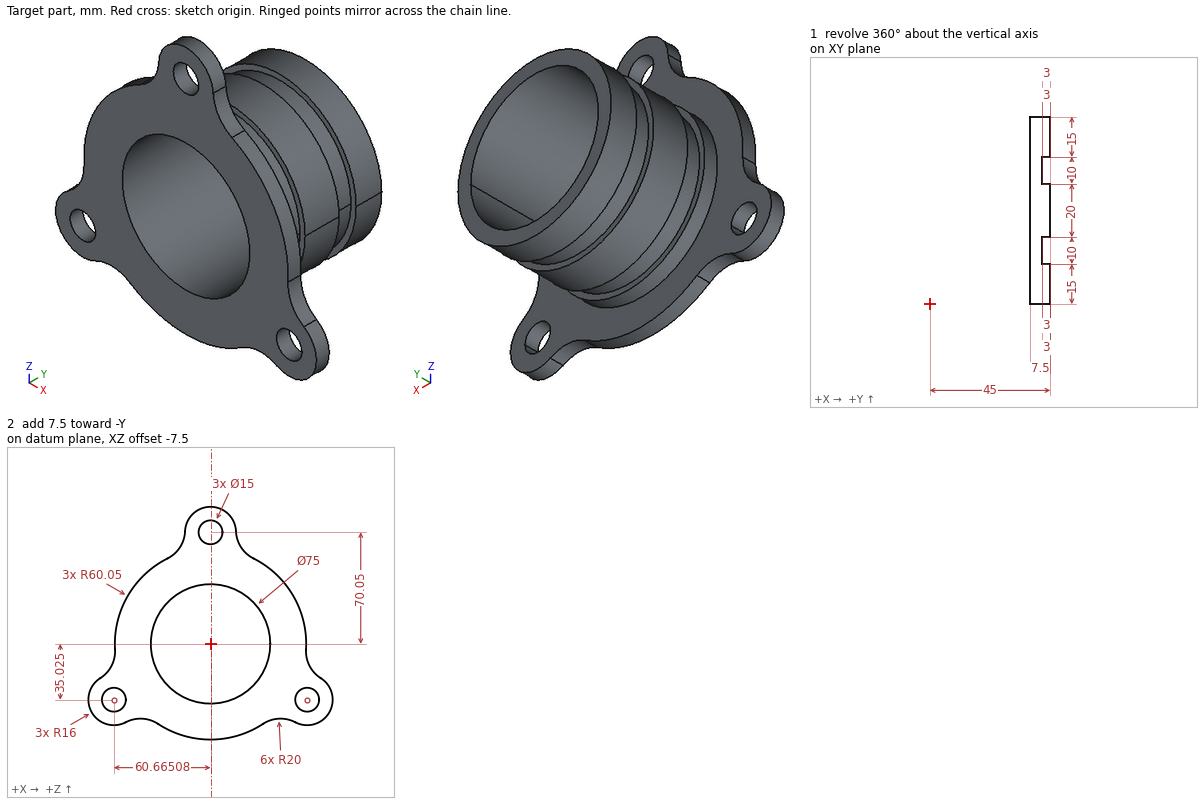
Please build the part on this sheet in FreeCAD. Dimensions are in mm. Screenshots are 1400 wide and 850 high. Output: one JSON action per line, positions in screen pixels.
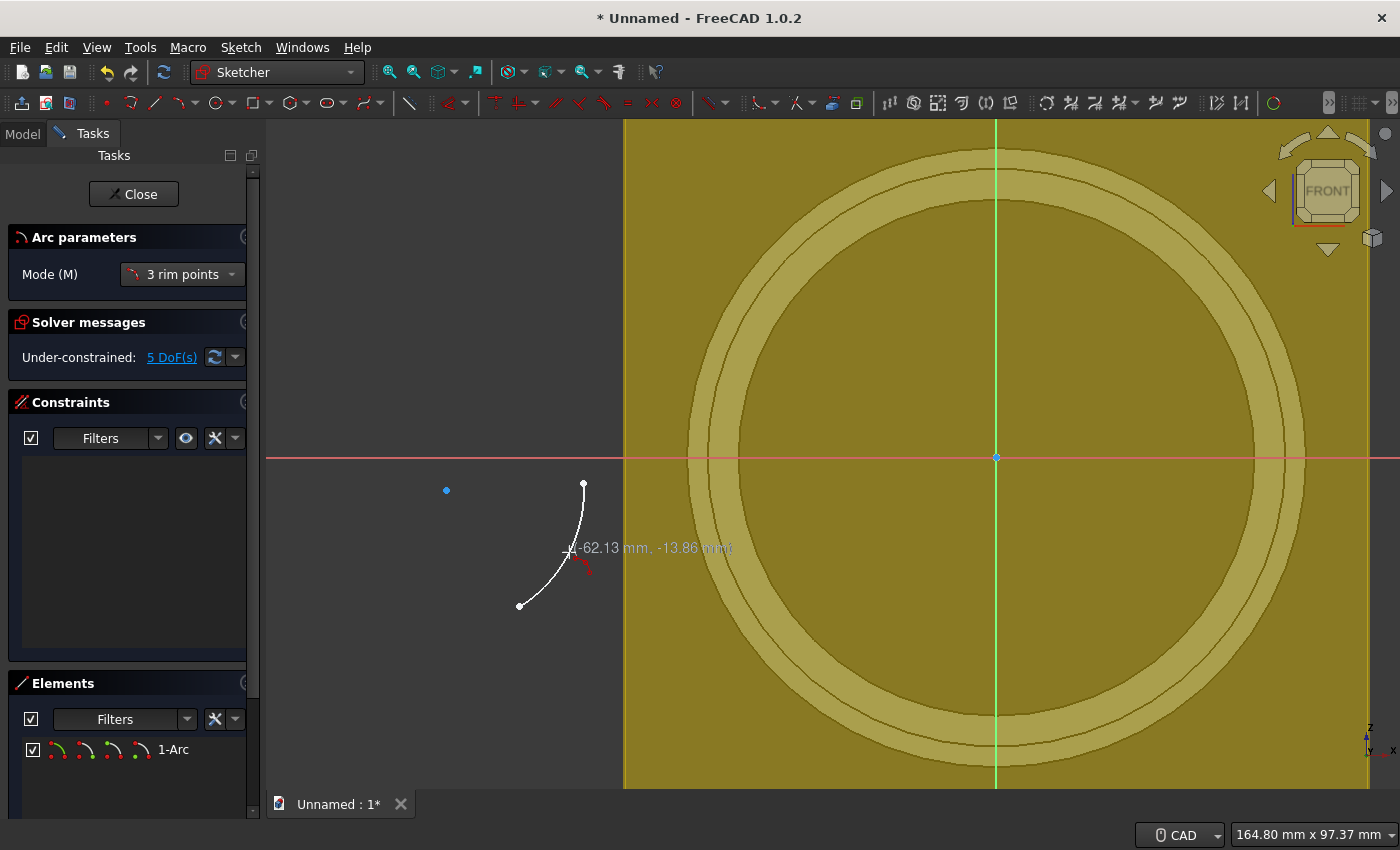
{"action": "left_click", "coordinate": [520, 607]}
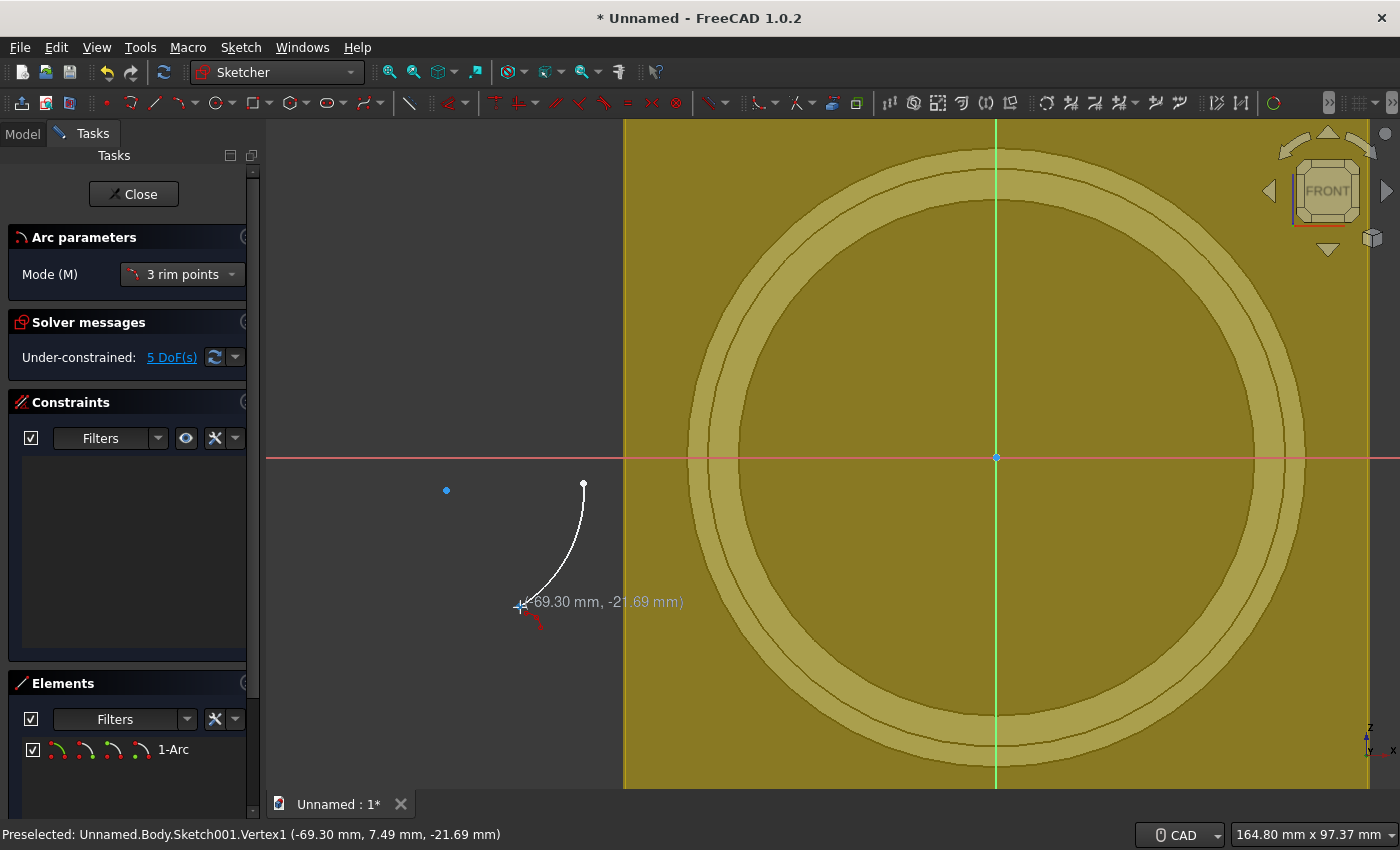
{"action": "scroll", "coordinate": [575, 524], "scroll_direction": "down", "scroll_amount": 4}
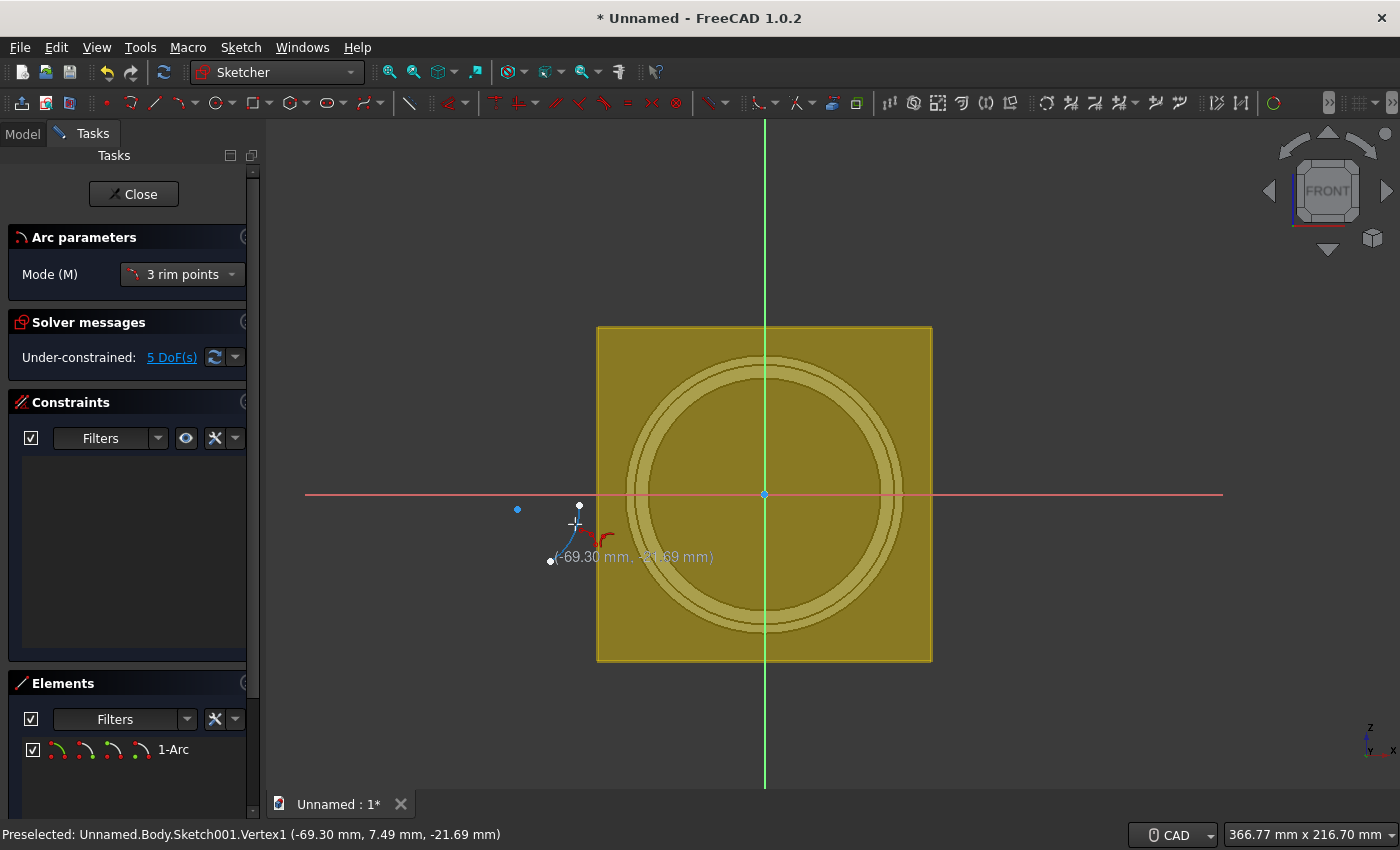
{"action": "left_click", "coordinate": [600, 647]}
{"action": "left_click", "coordinate": [534, 628]}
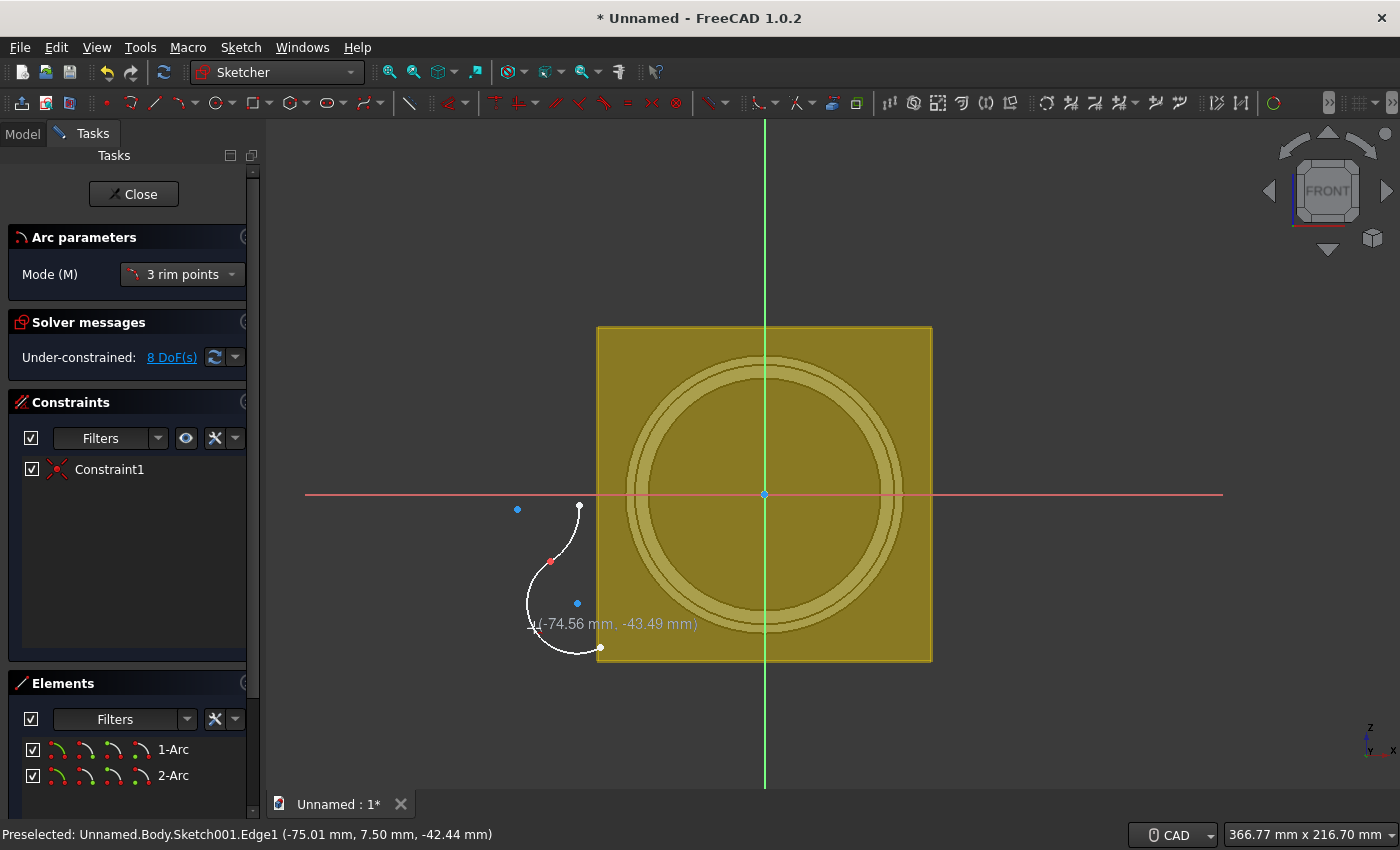
{"action": "left_click", "coordinate": [600, 648]}
{"action": "left_click", "coordinate": [663, 650]}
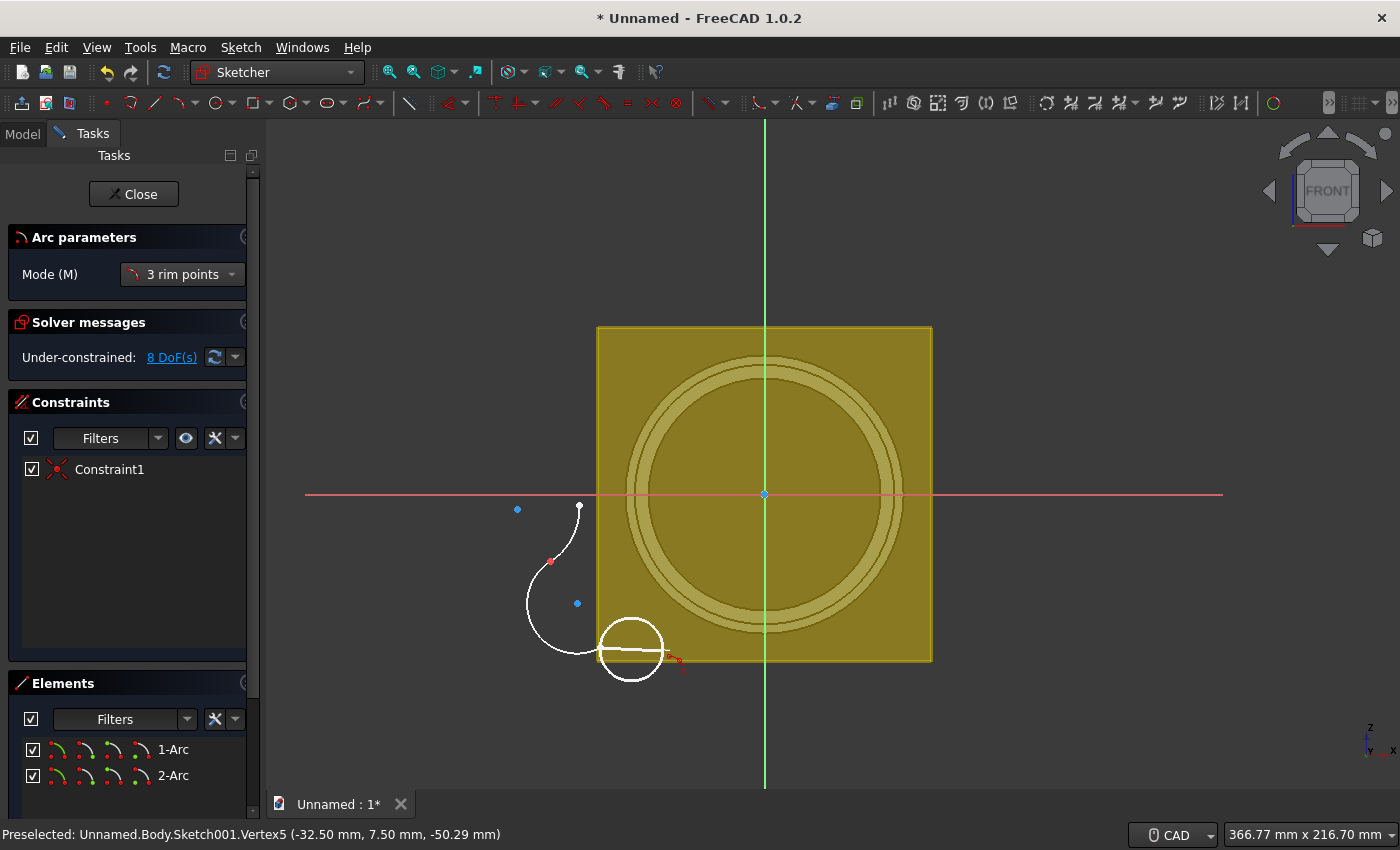
{"action": "scroll", "coordinate": [632, 640], "scroll_direction": "up", "scroll_amount": 4}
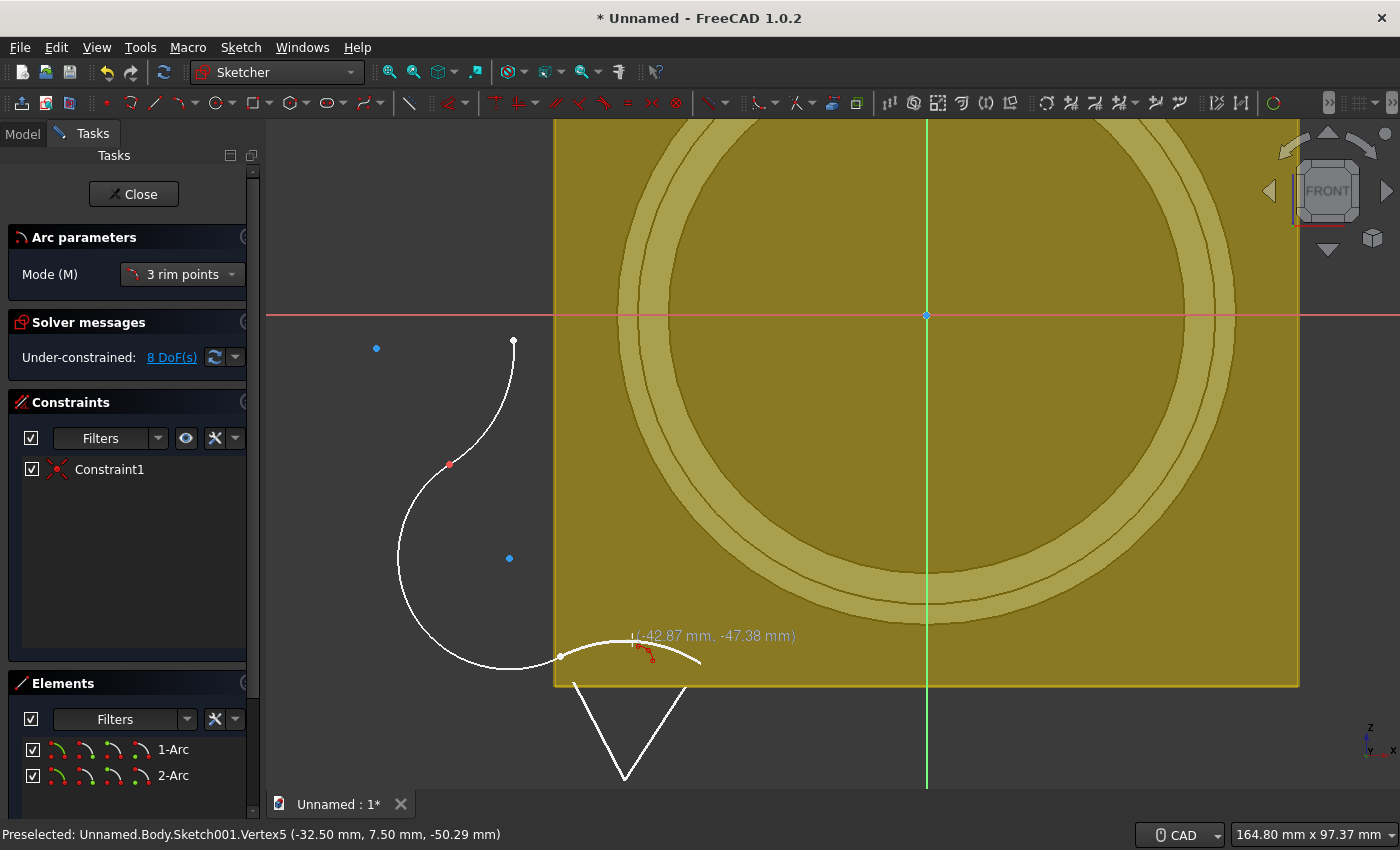
{"action": "left_click", "coordinate": [631, 638]}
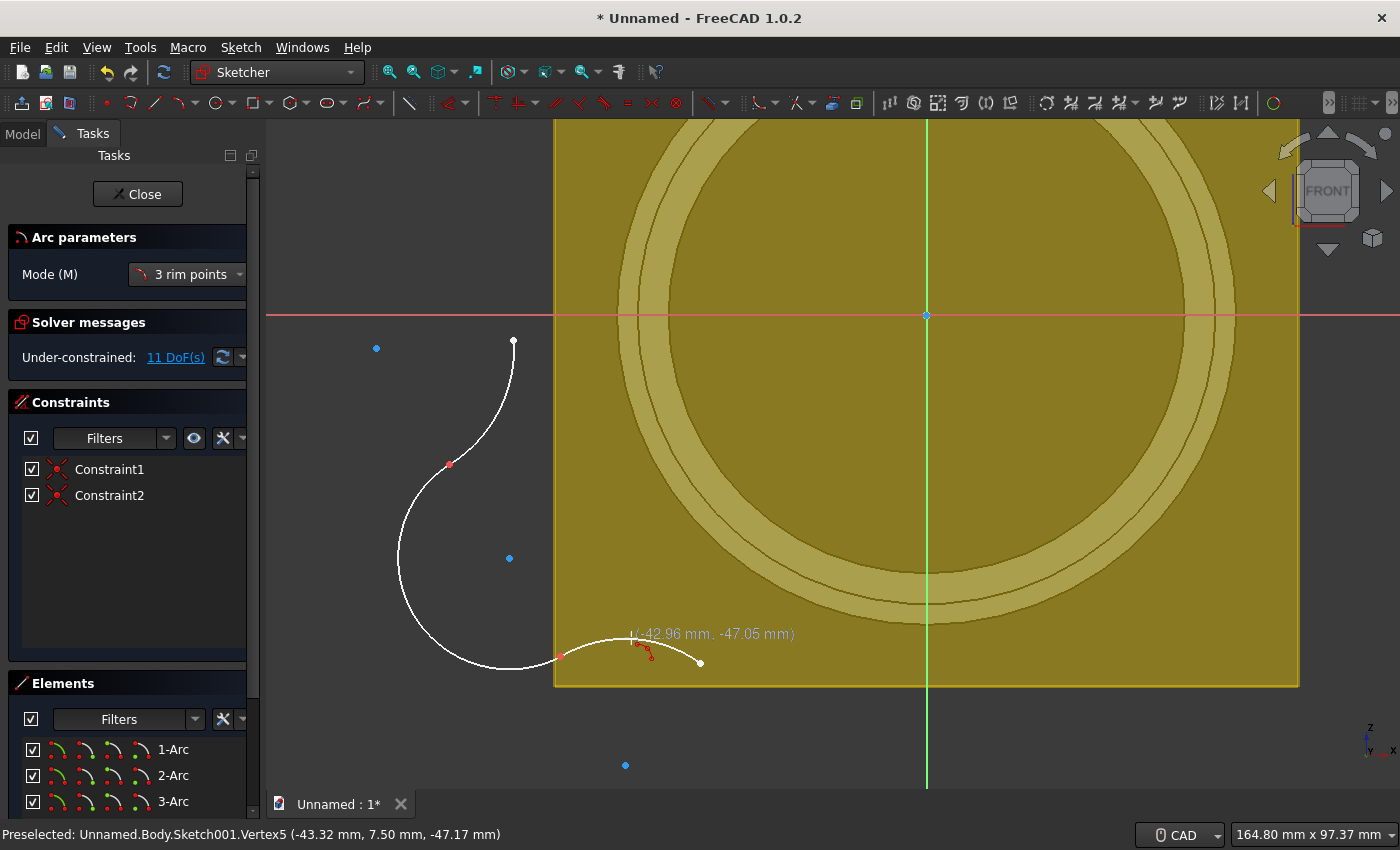
{"action": "left_click", "coordinate": [701, 664]}
{"action": "left_click", "coordinate": [1153, 661]}
{"action": "left_click", "coordinate": [879, 726]}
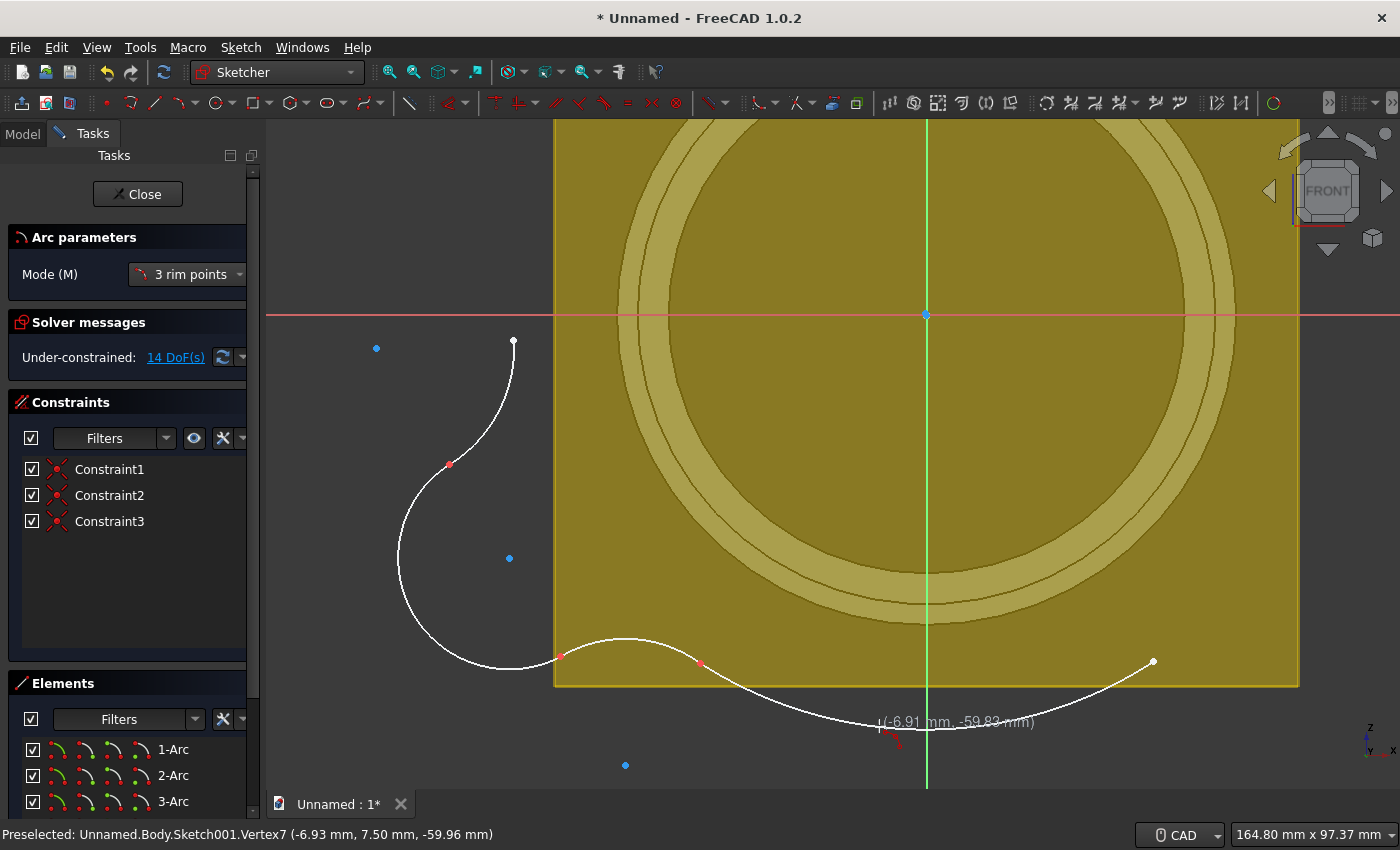
{"action": "left_click", "coordinate": [1153, 662]}